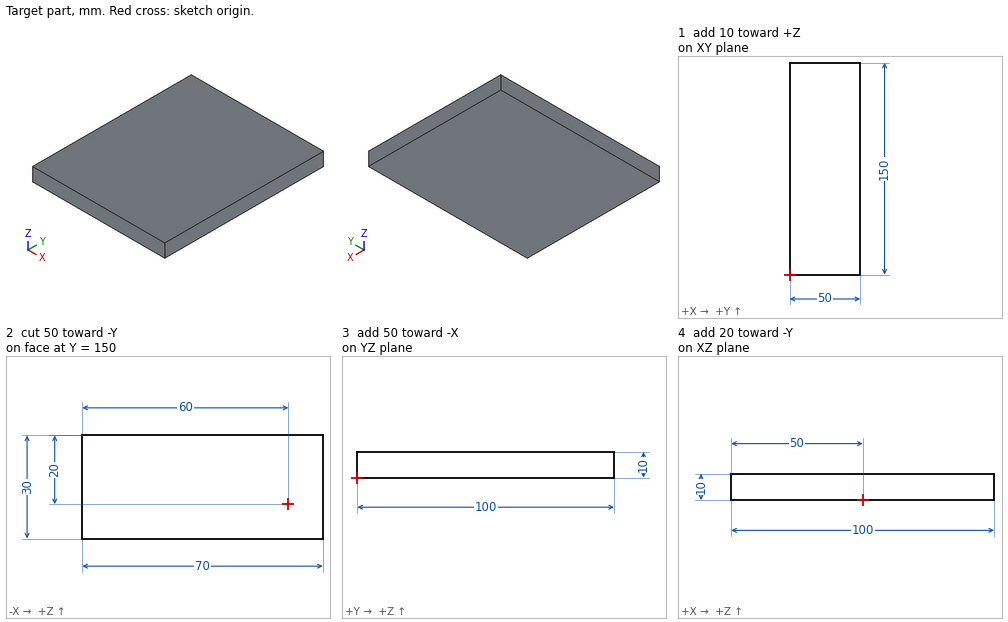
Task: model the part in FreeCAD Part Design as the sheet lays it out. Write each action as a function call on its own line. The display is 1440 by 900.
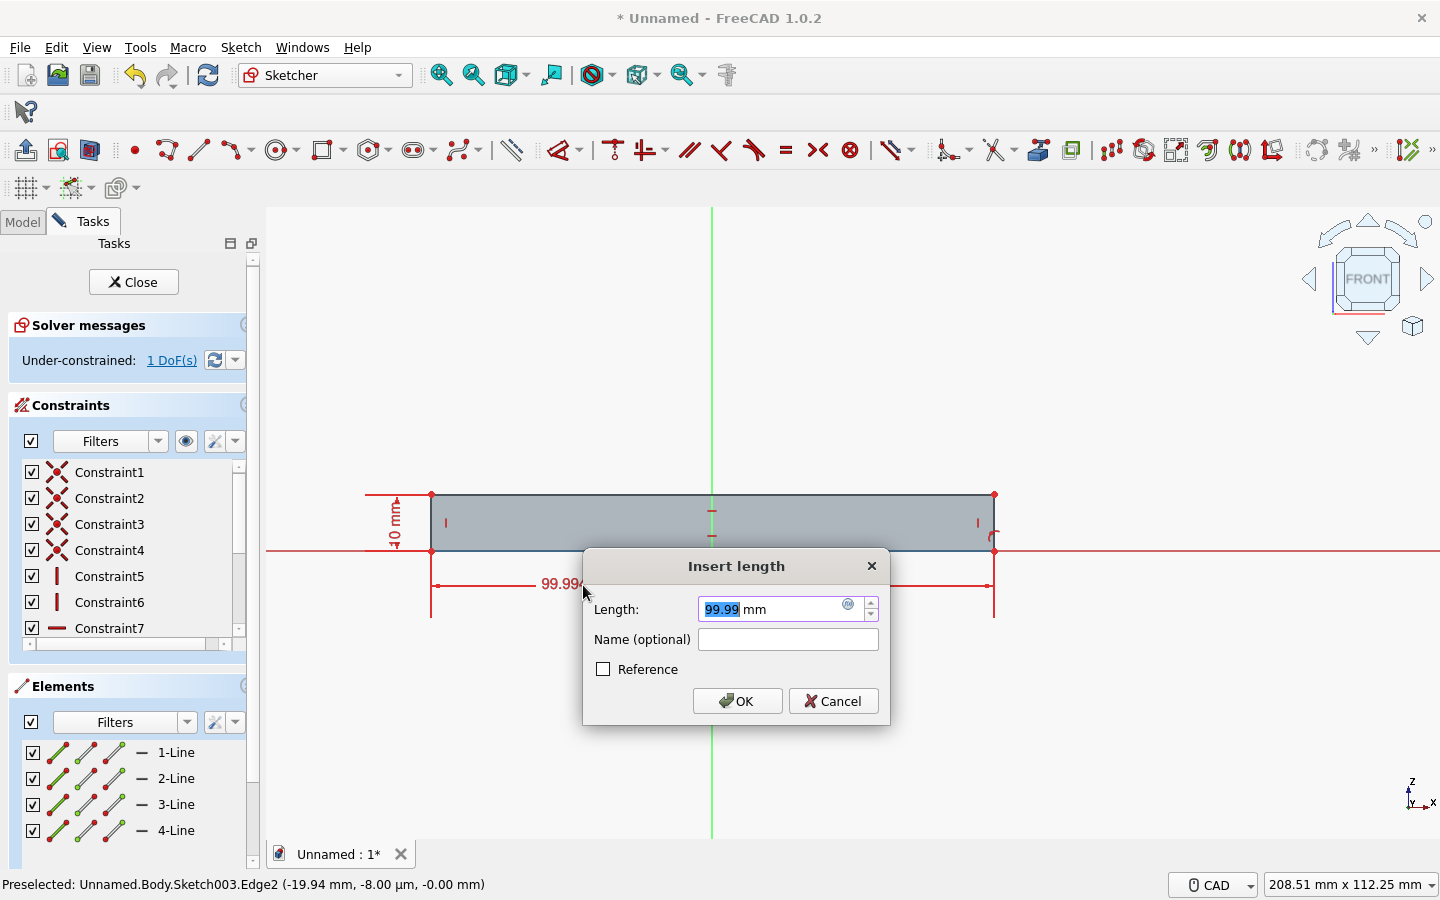
text(100)
key(Return)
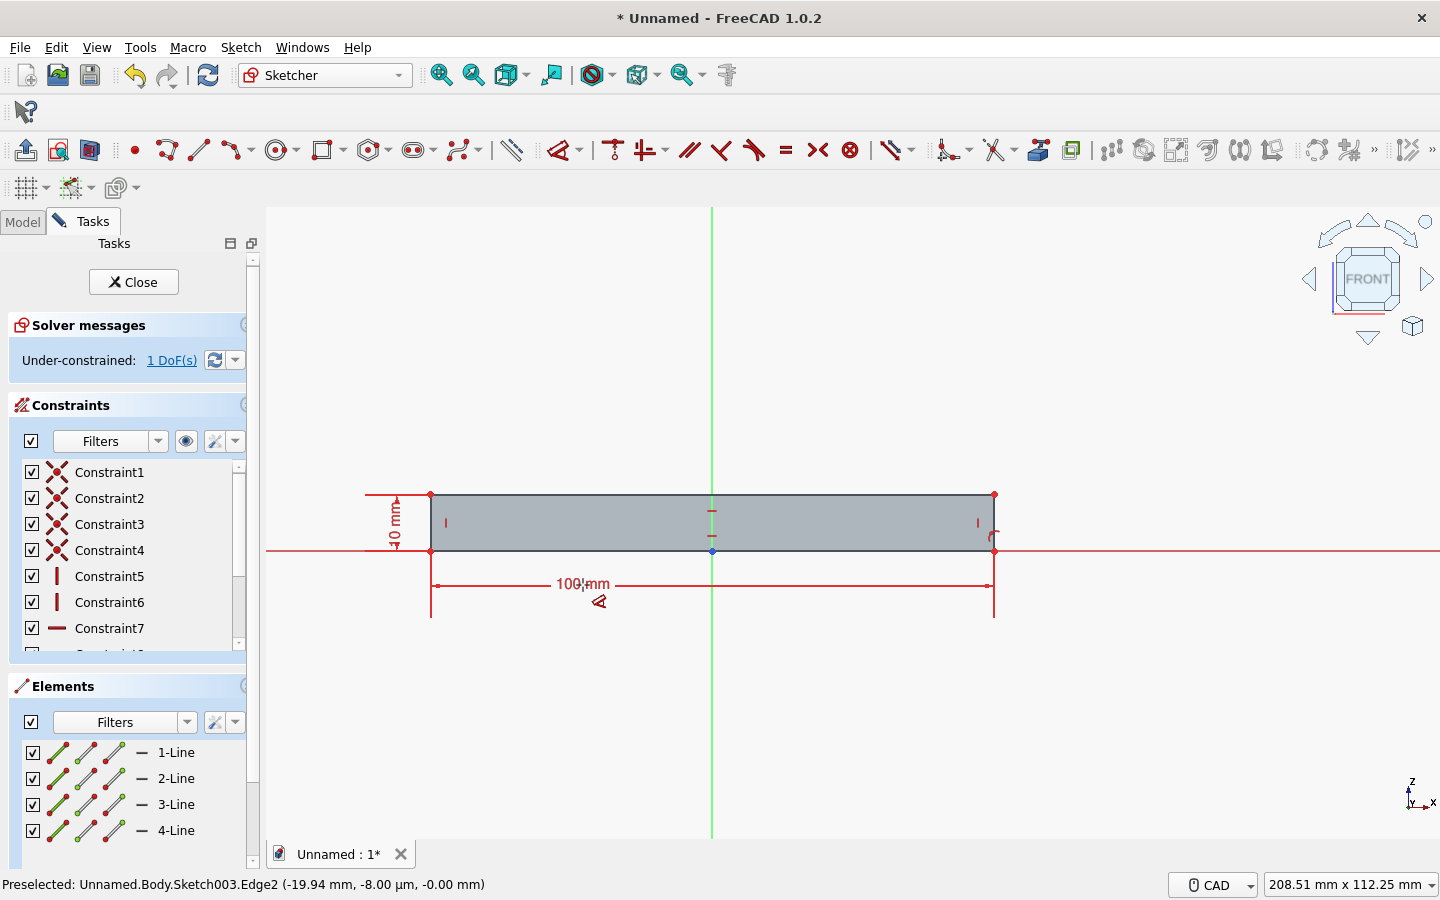
click(431, 495)
click(507, 585)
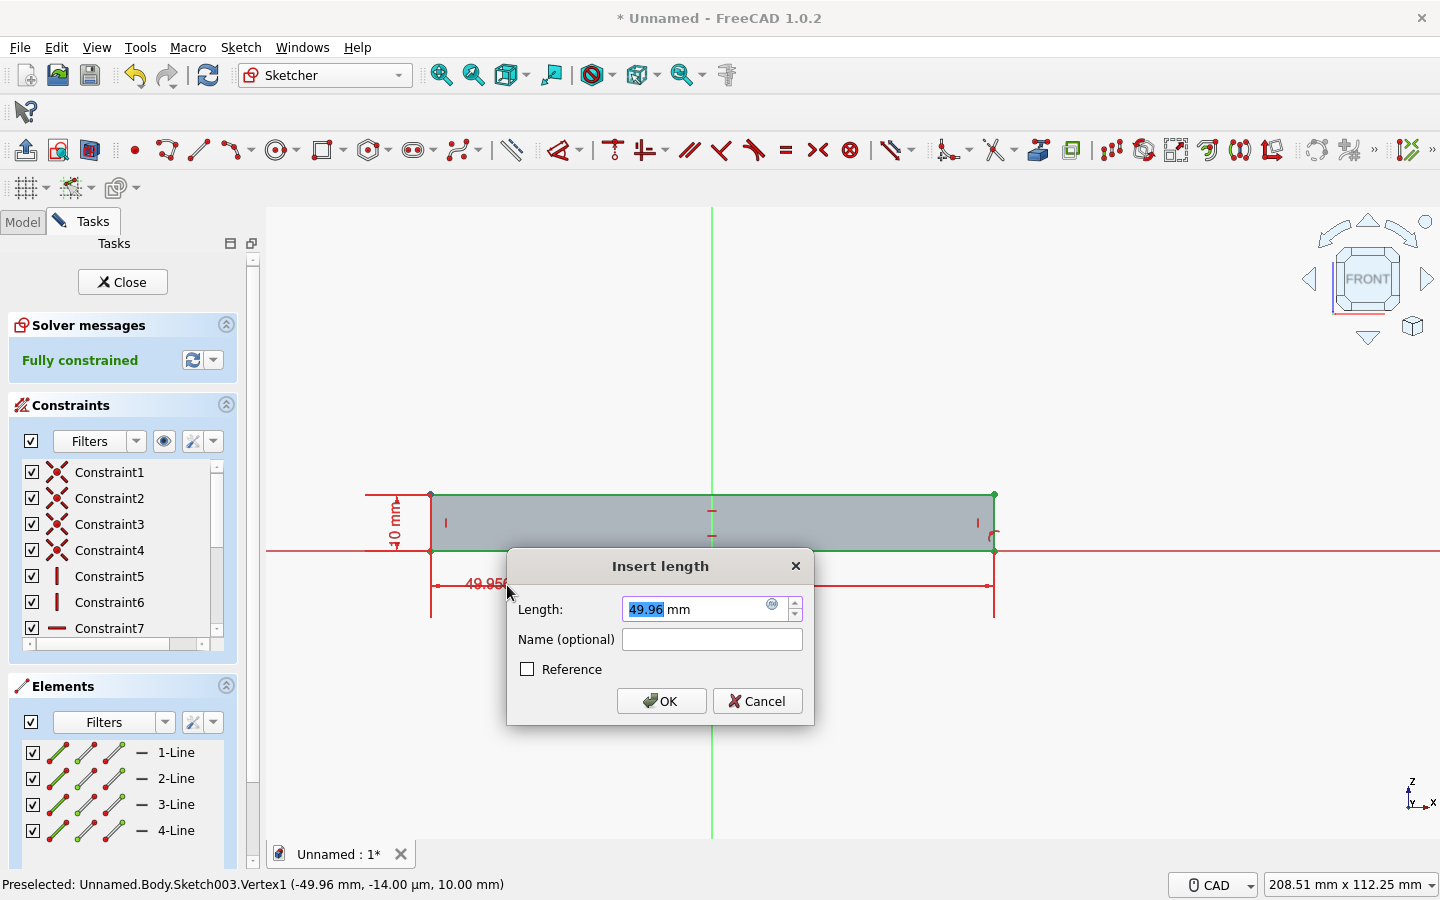
text(50)
key(Return)
key(Escape)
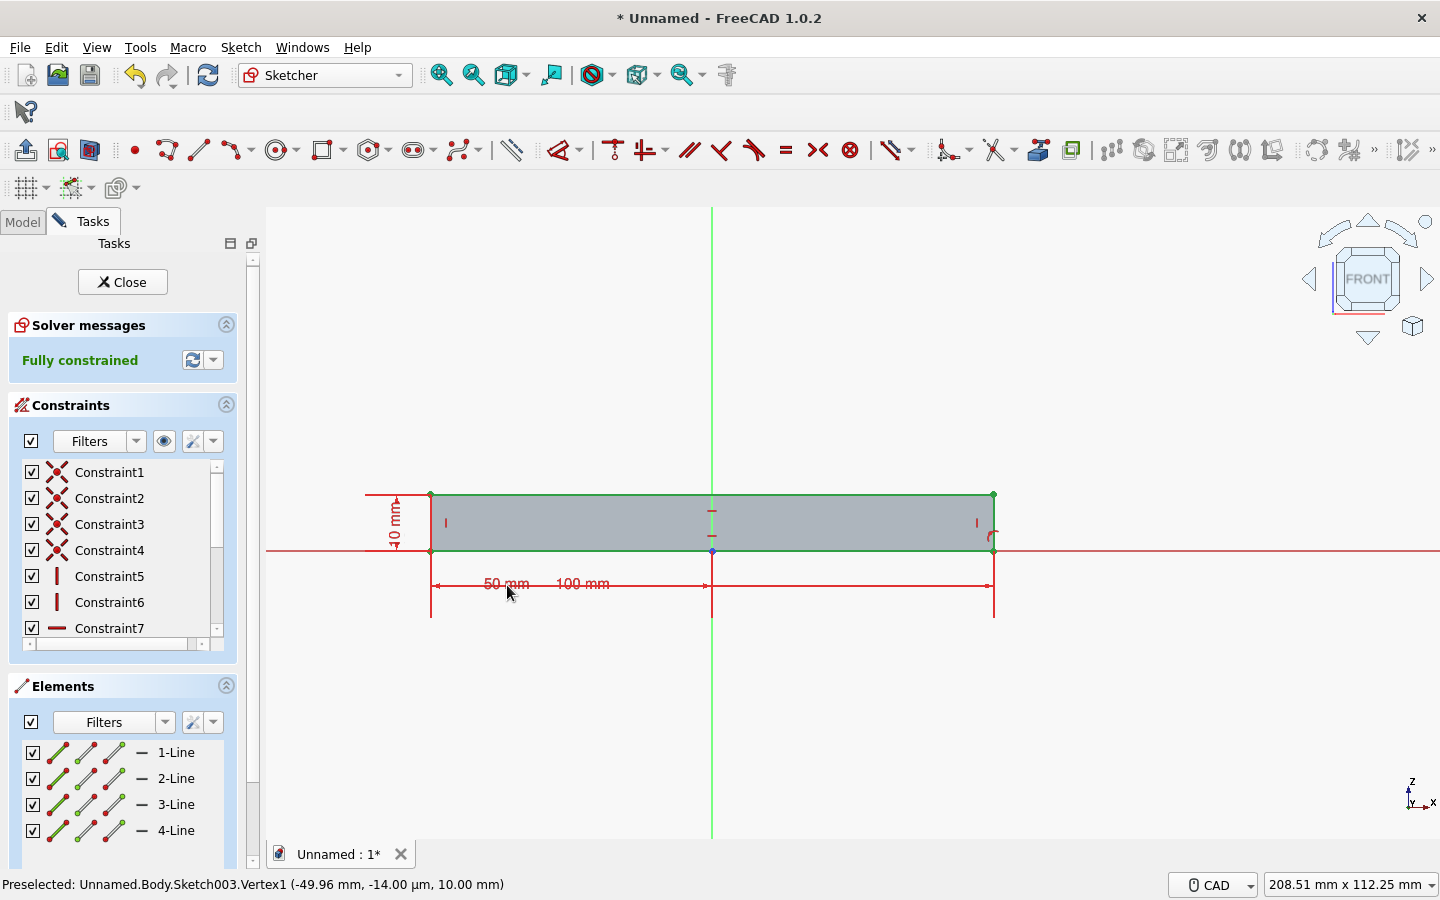
click(123, 282)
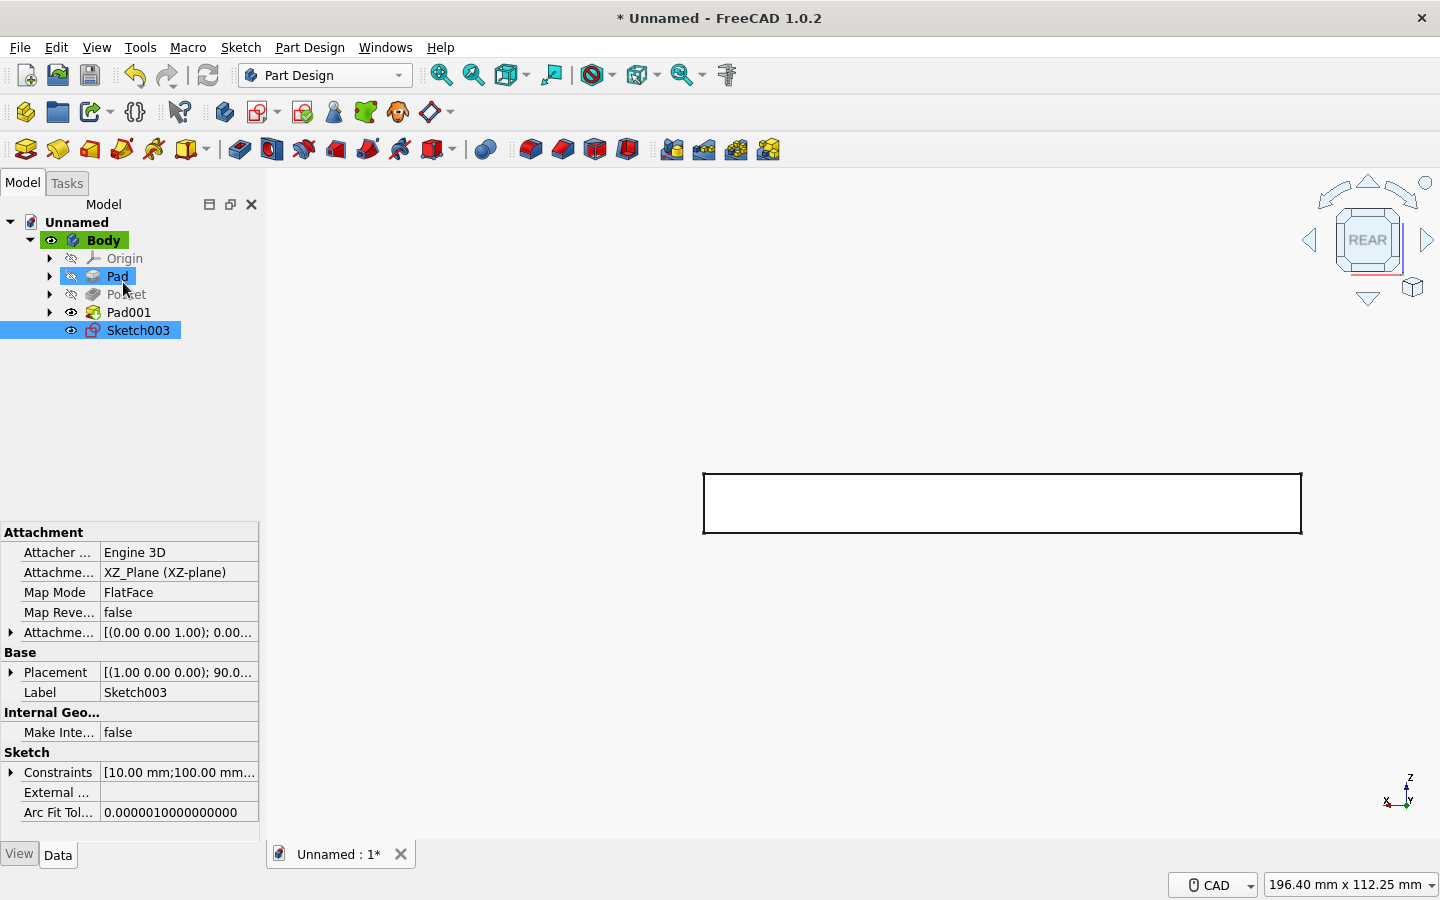
click(26, 150)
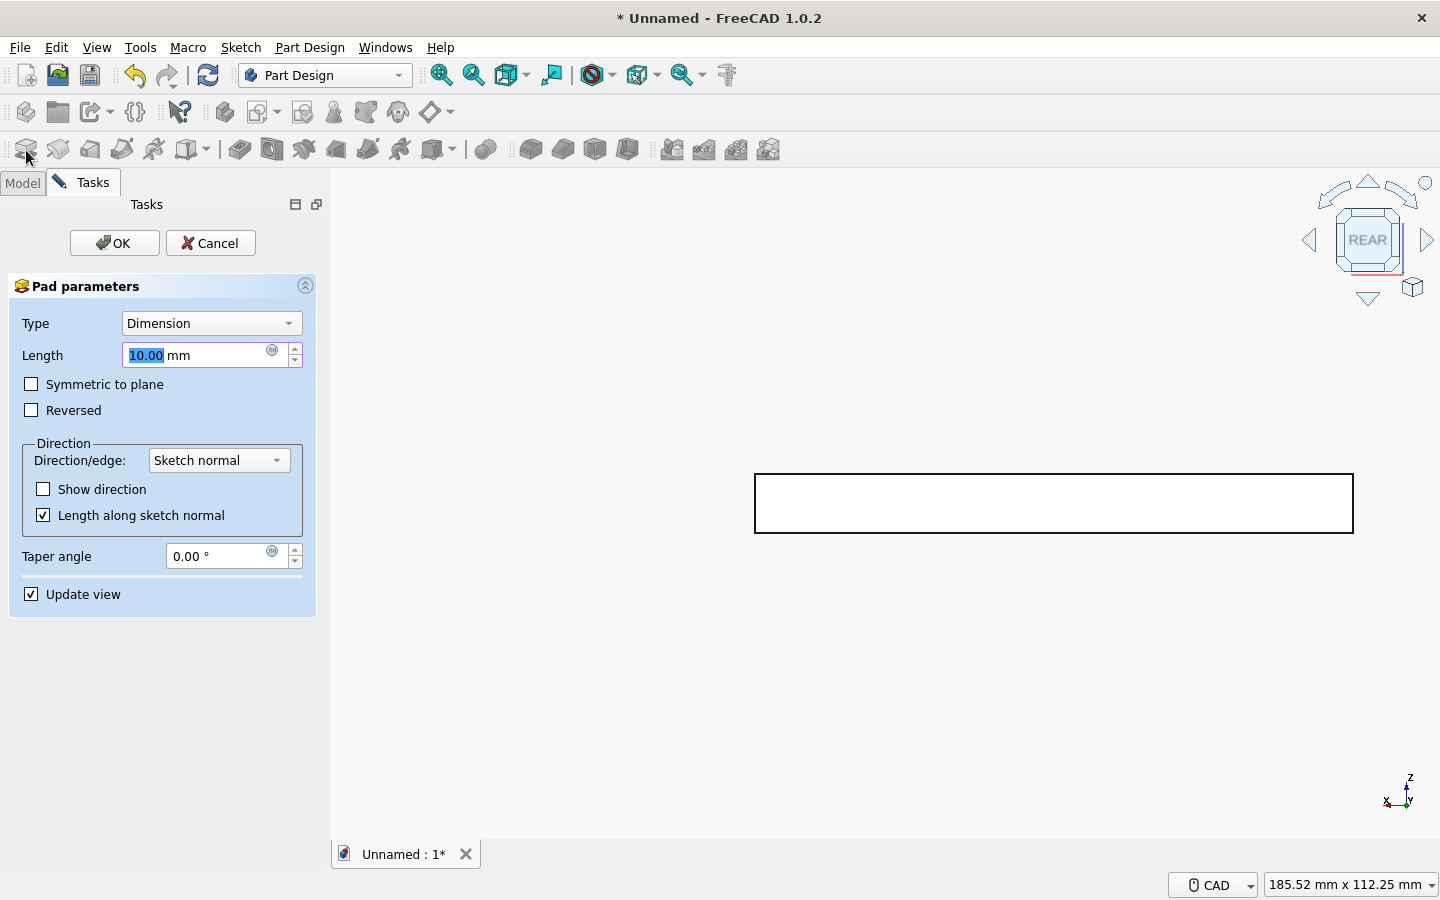
text(20)
key(Tab)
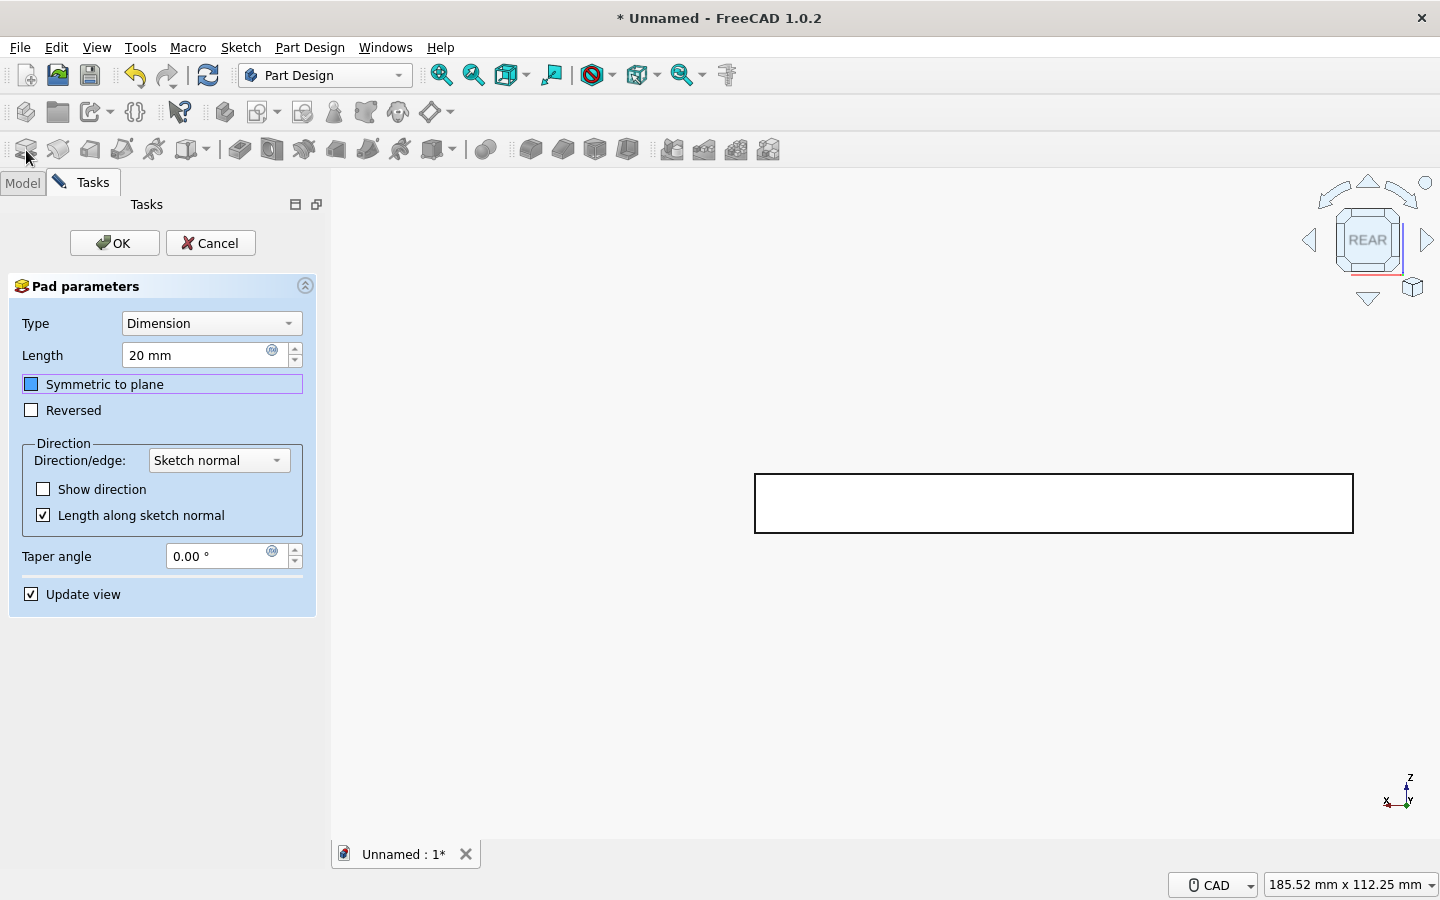
click(115, 243)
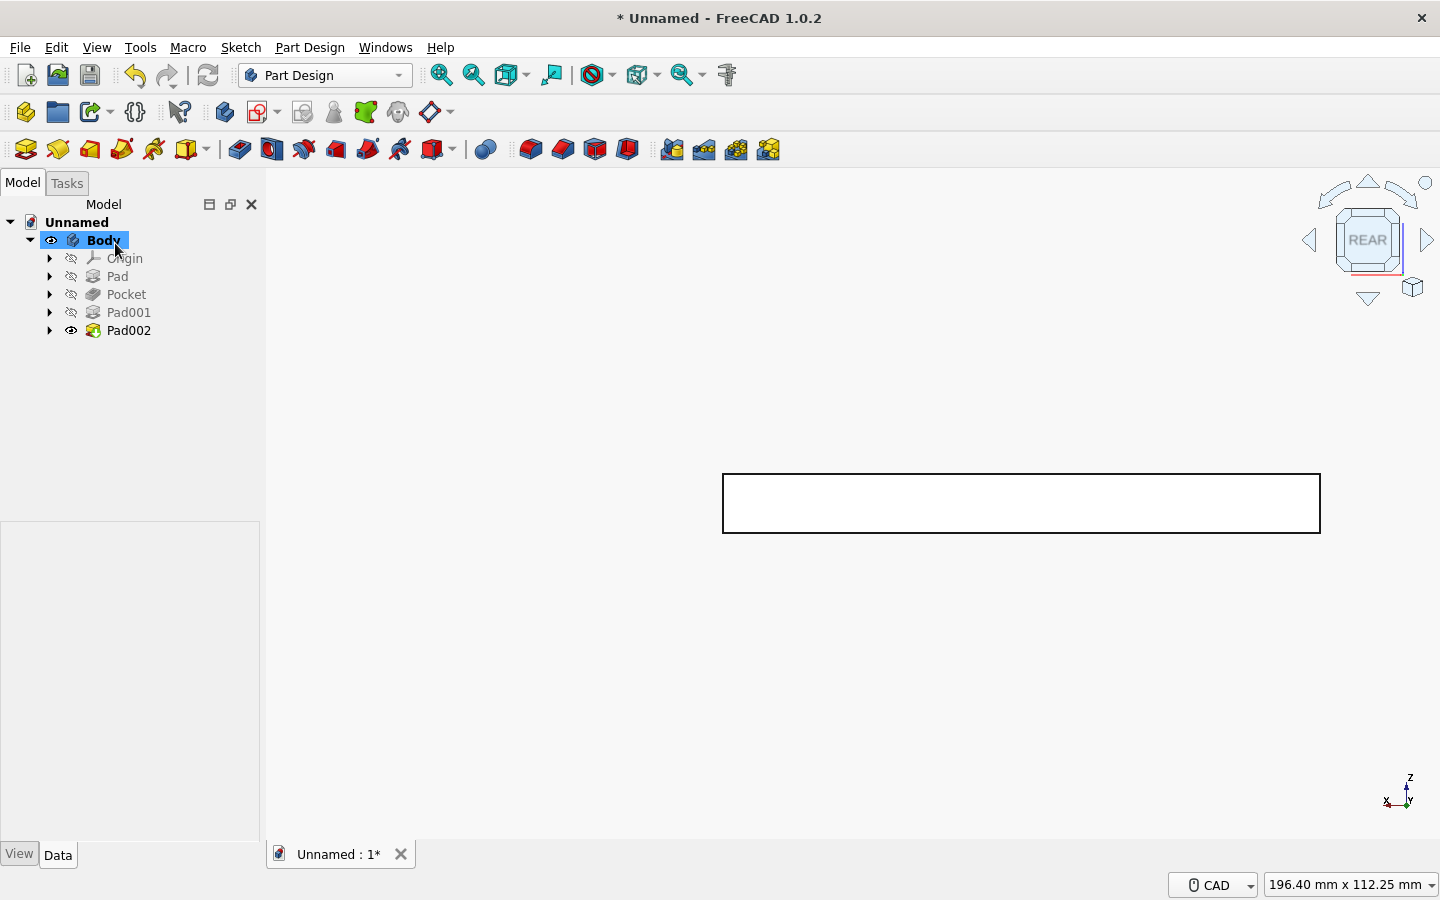
key(0)